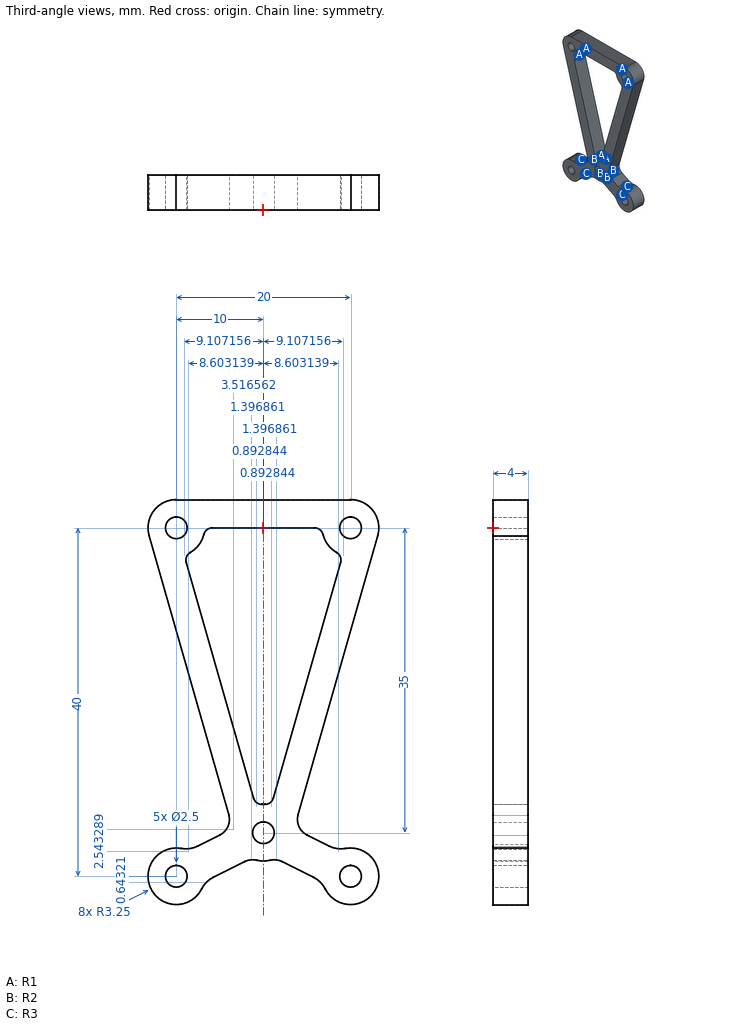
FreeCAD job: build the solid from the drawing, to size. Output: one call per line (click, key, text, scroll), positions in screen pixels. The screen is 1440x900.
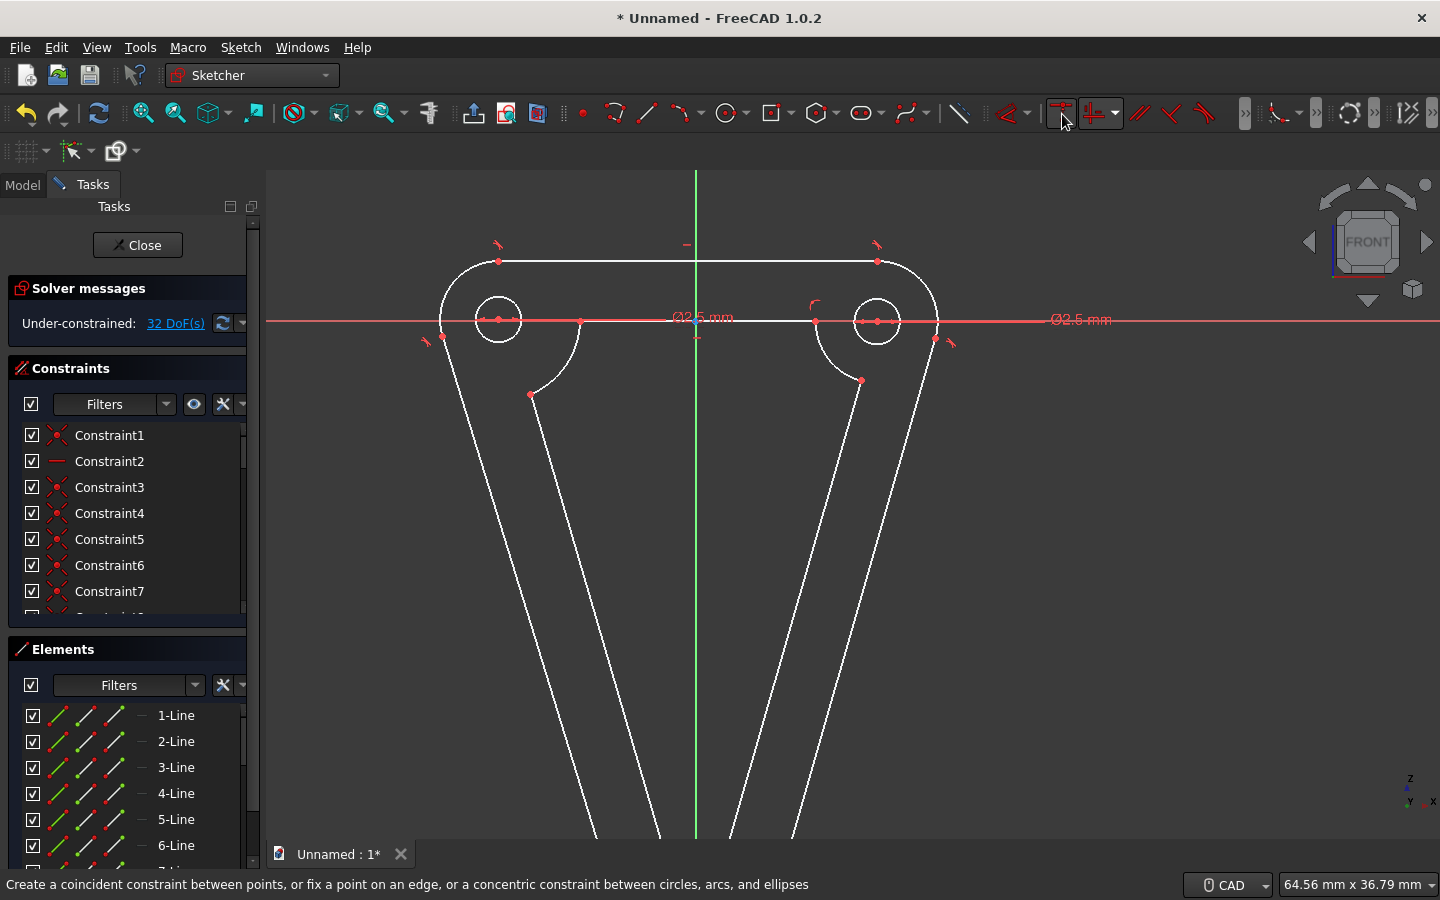
scroll(893, 305, down, 3)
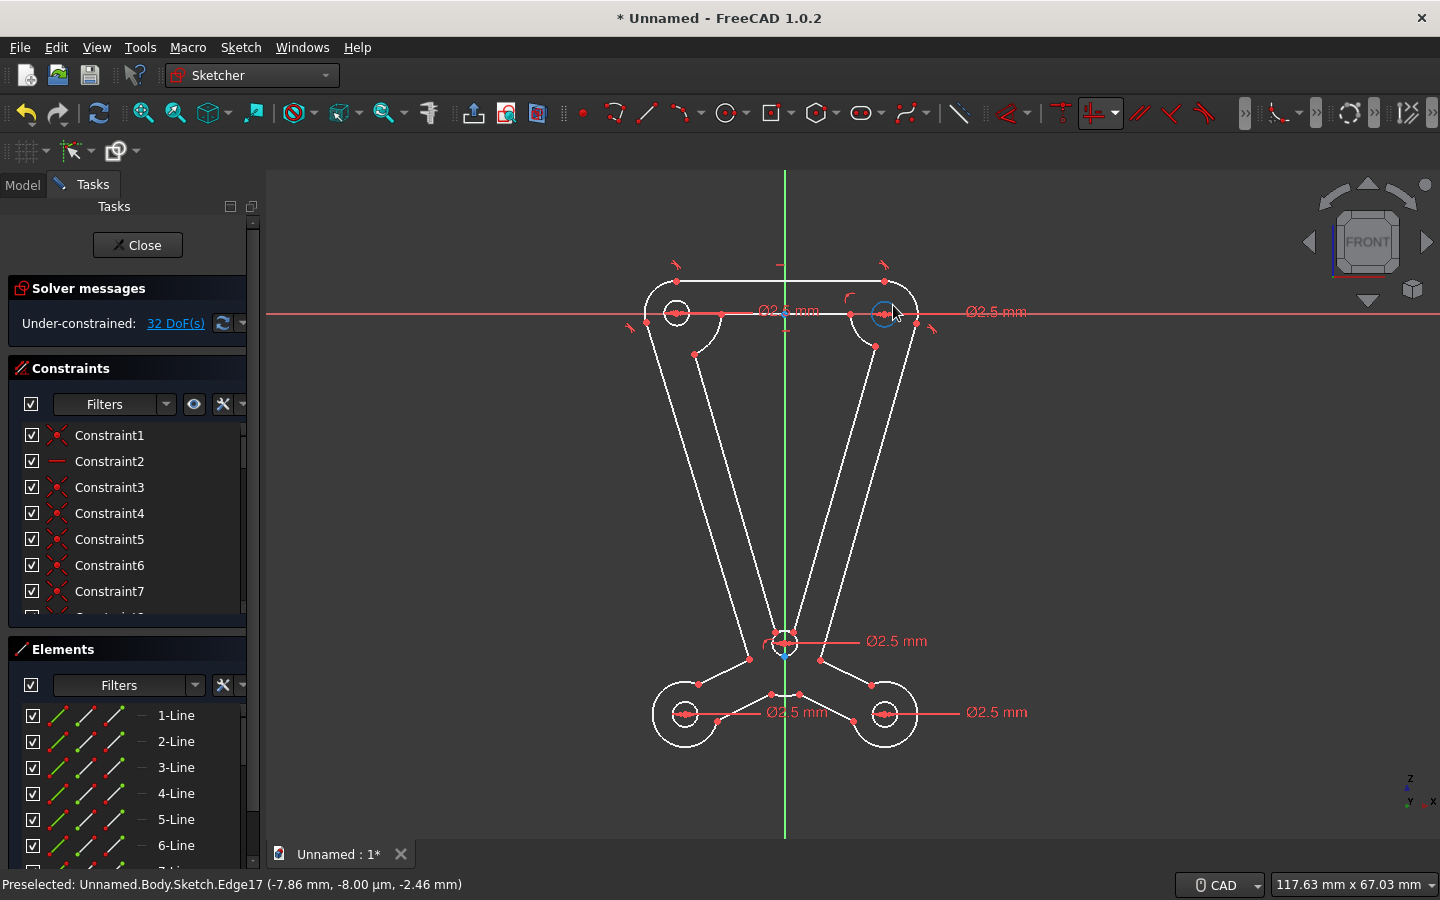
scroll(776, 652, up, 3)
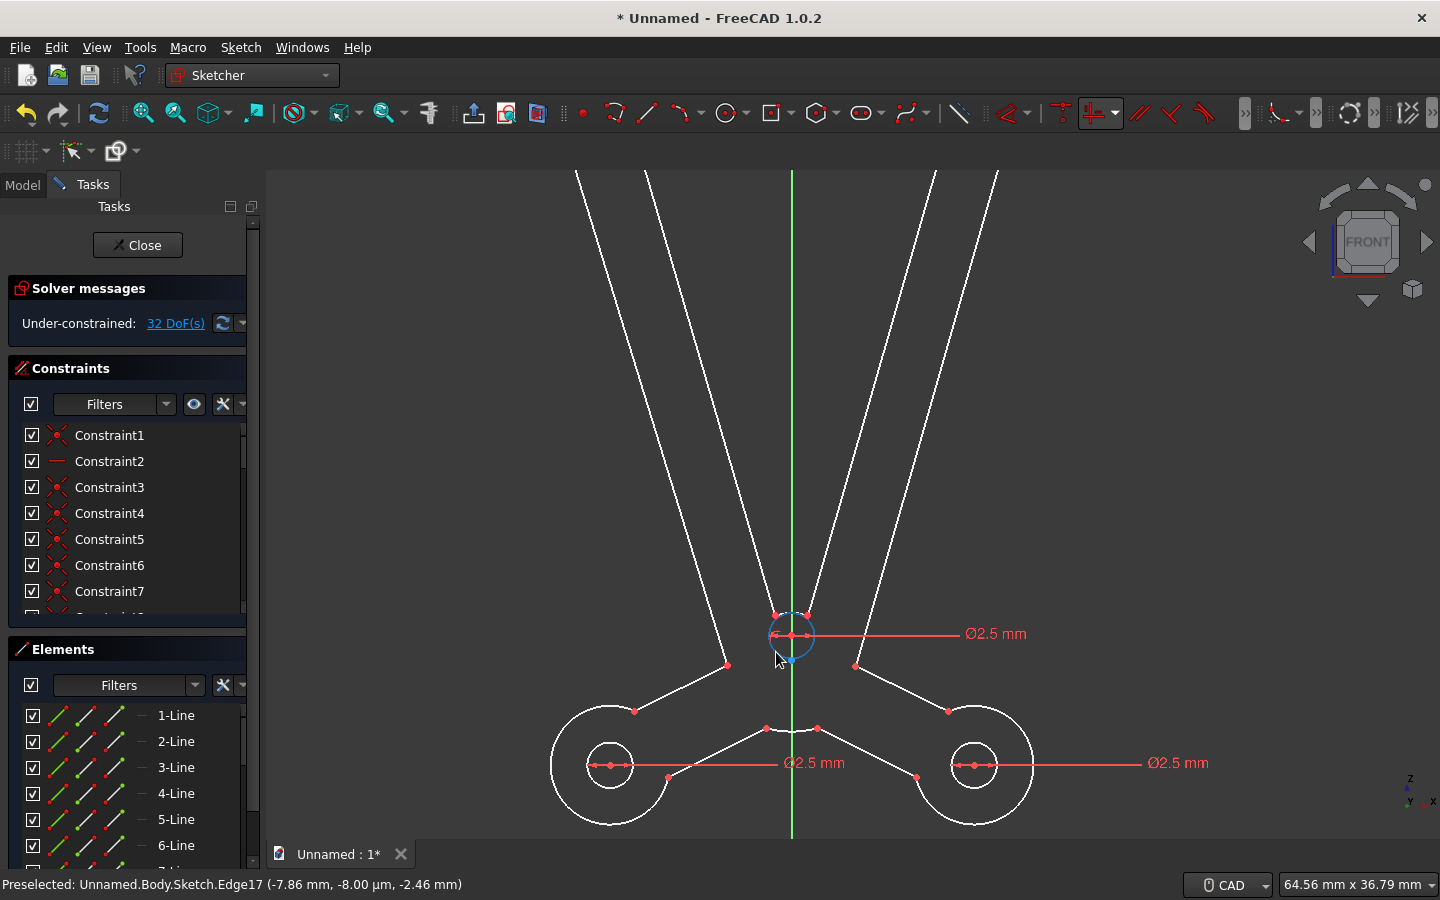
click(776, 652)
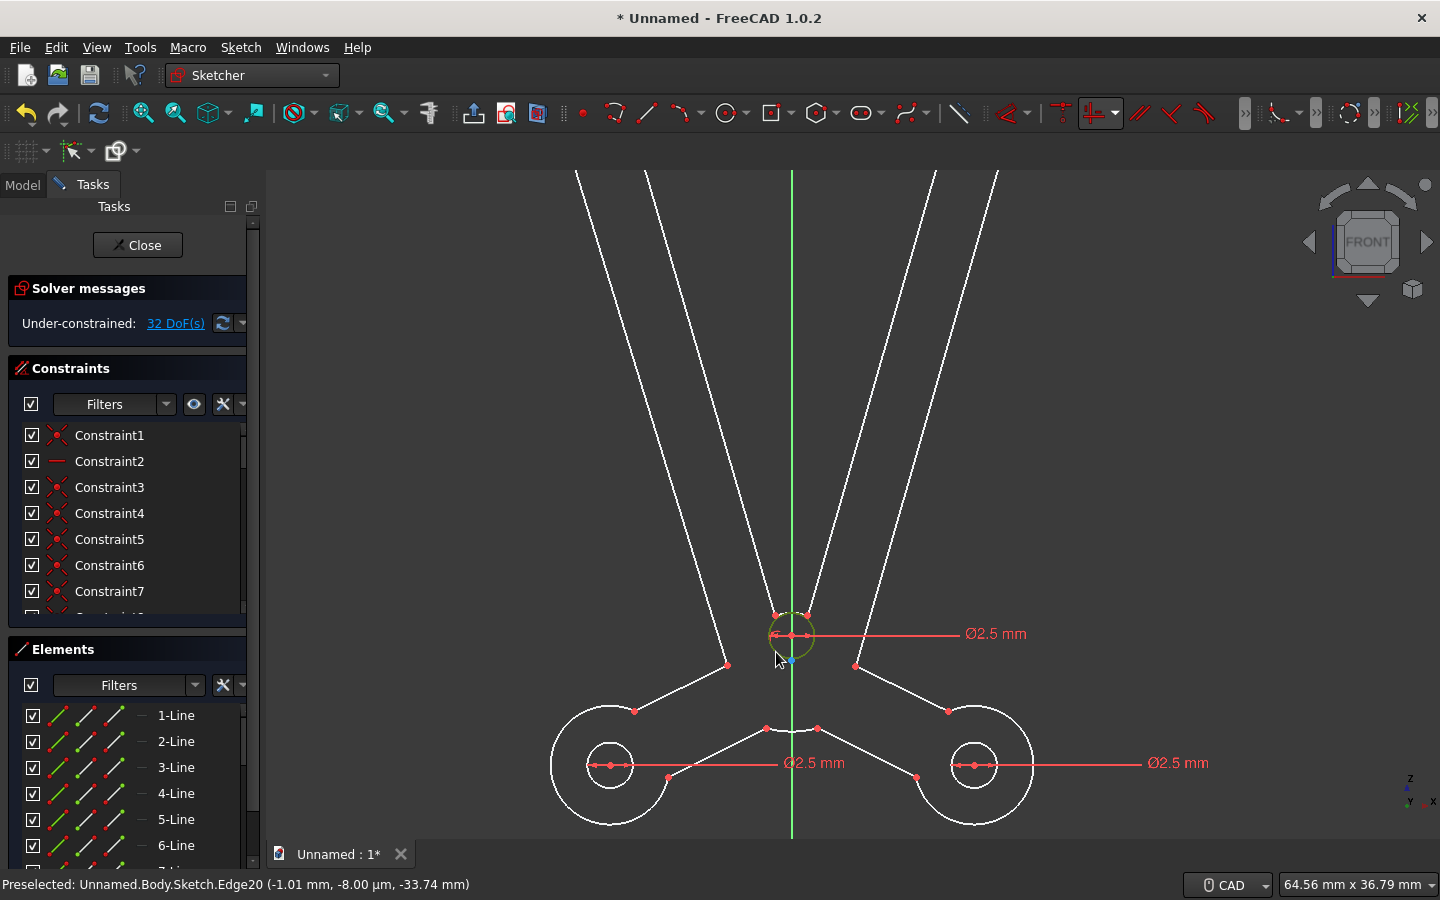
scroll(782, 614, up, 11)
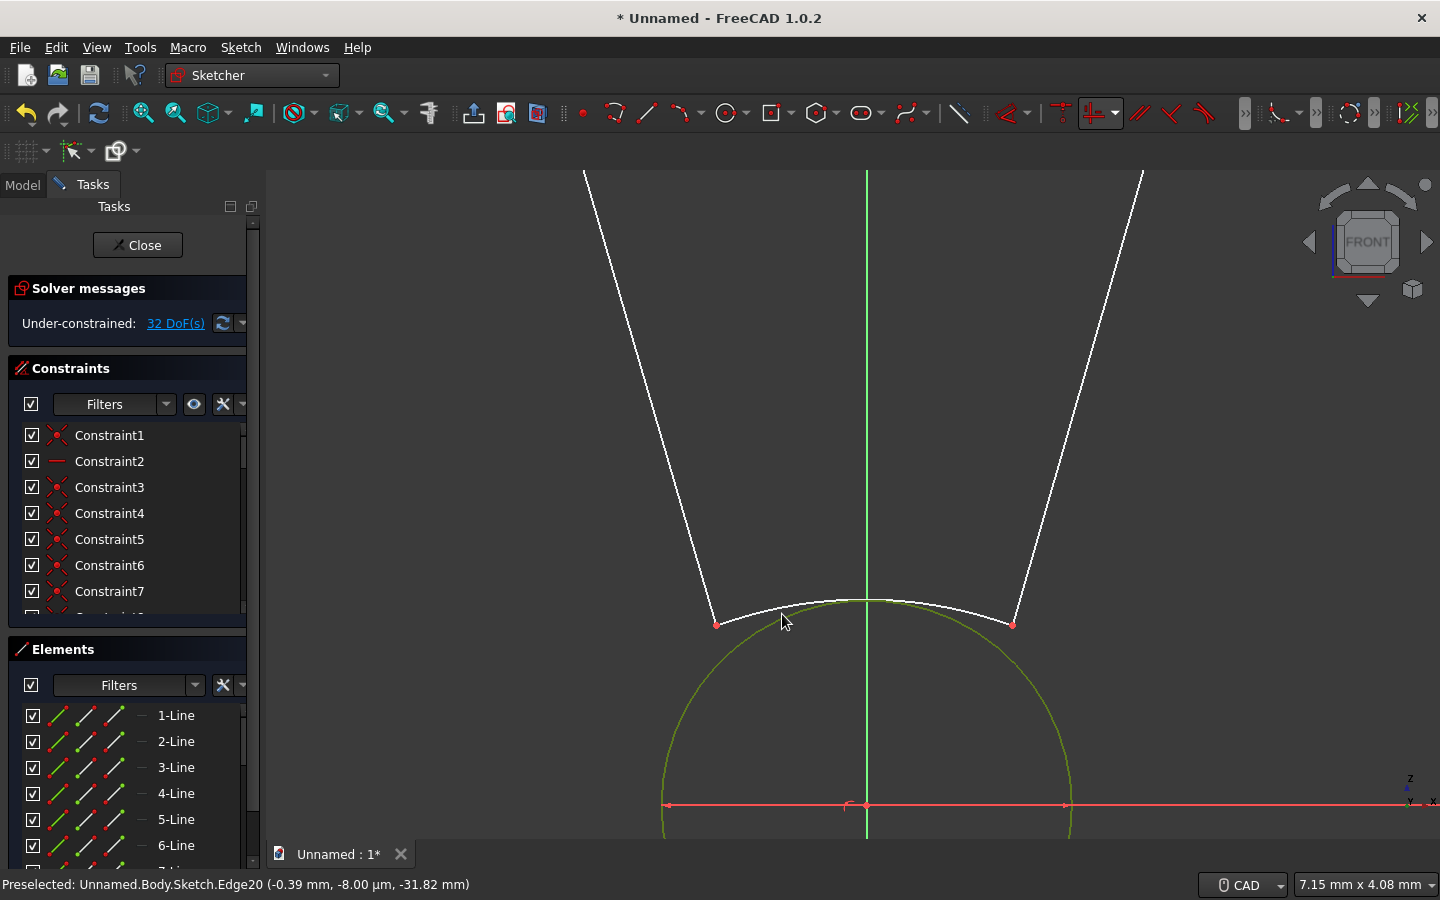
click(774, 609)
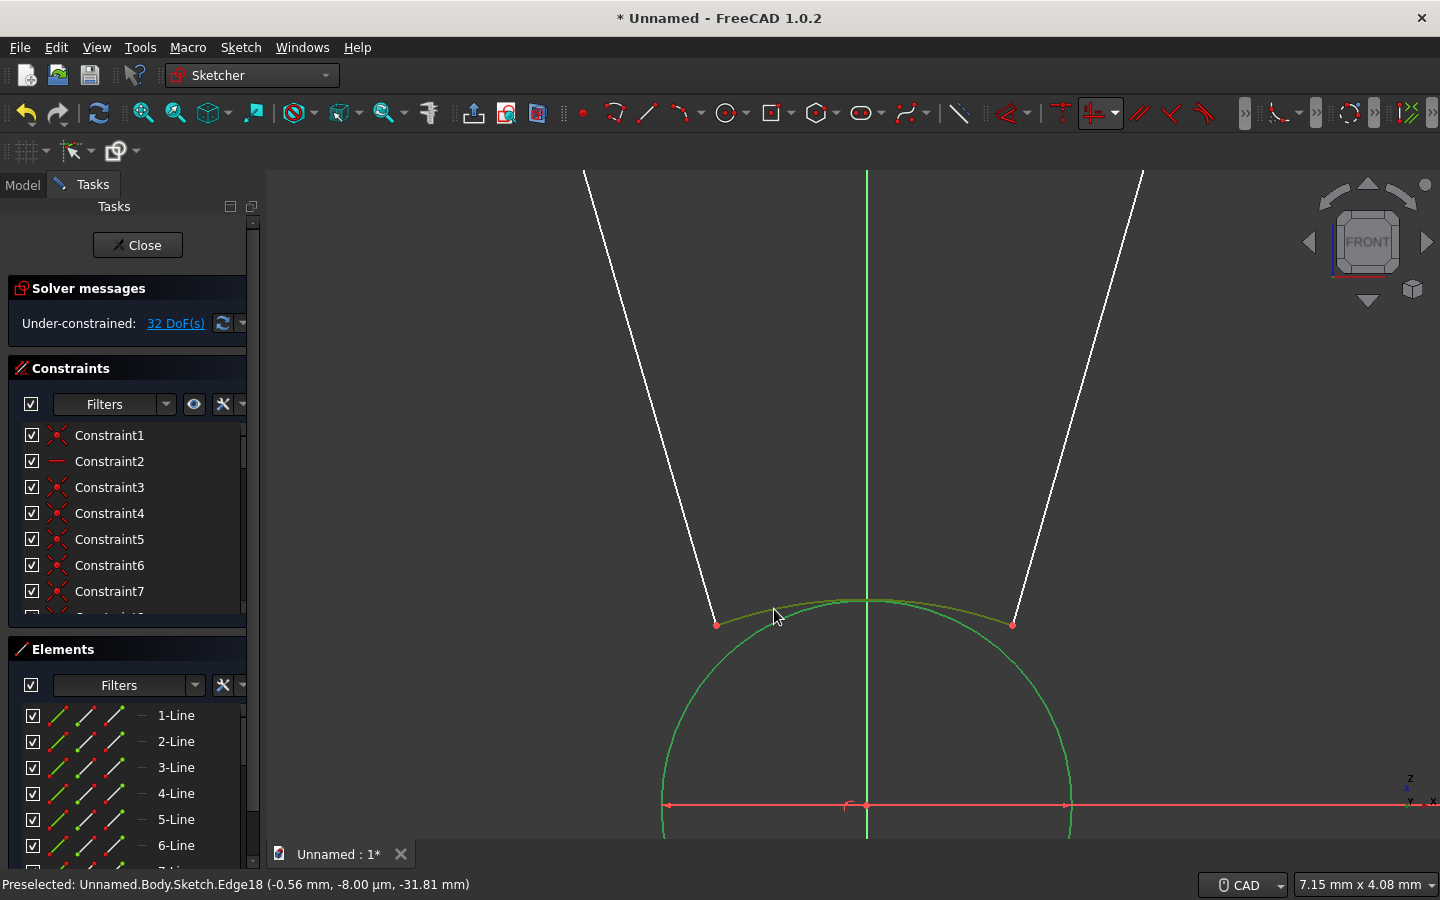
click(1062, 114)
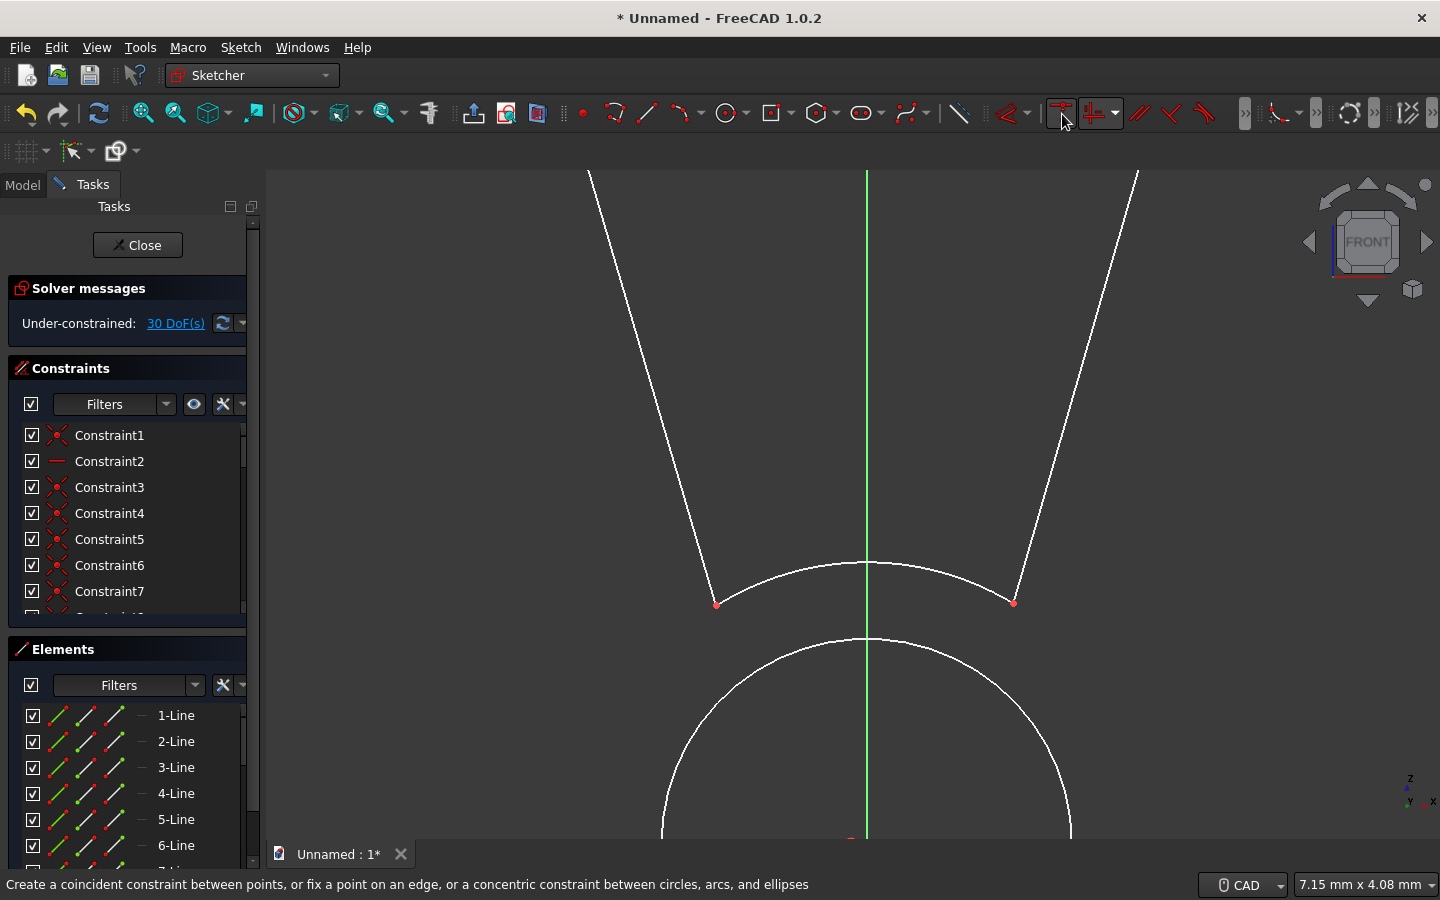
scroll(779, 633, down, 14)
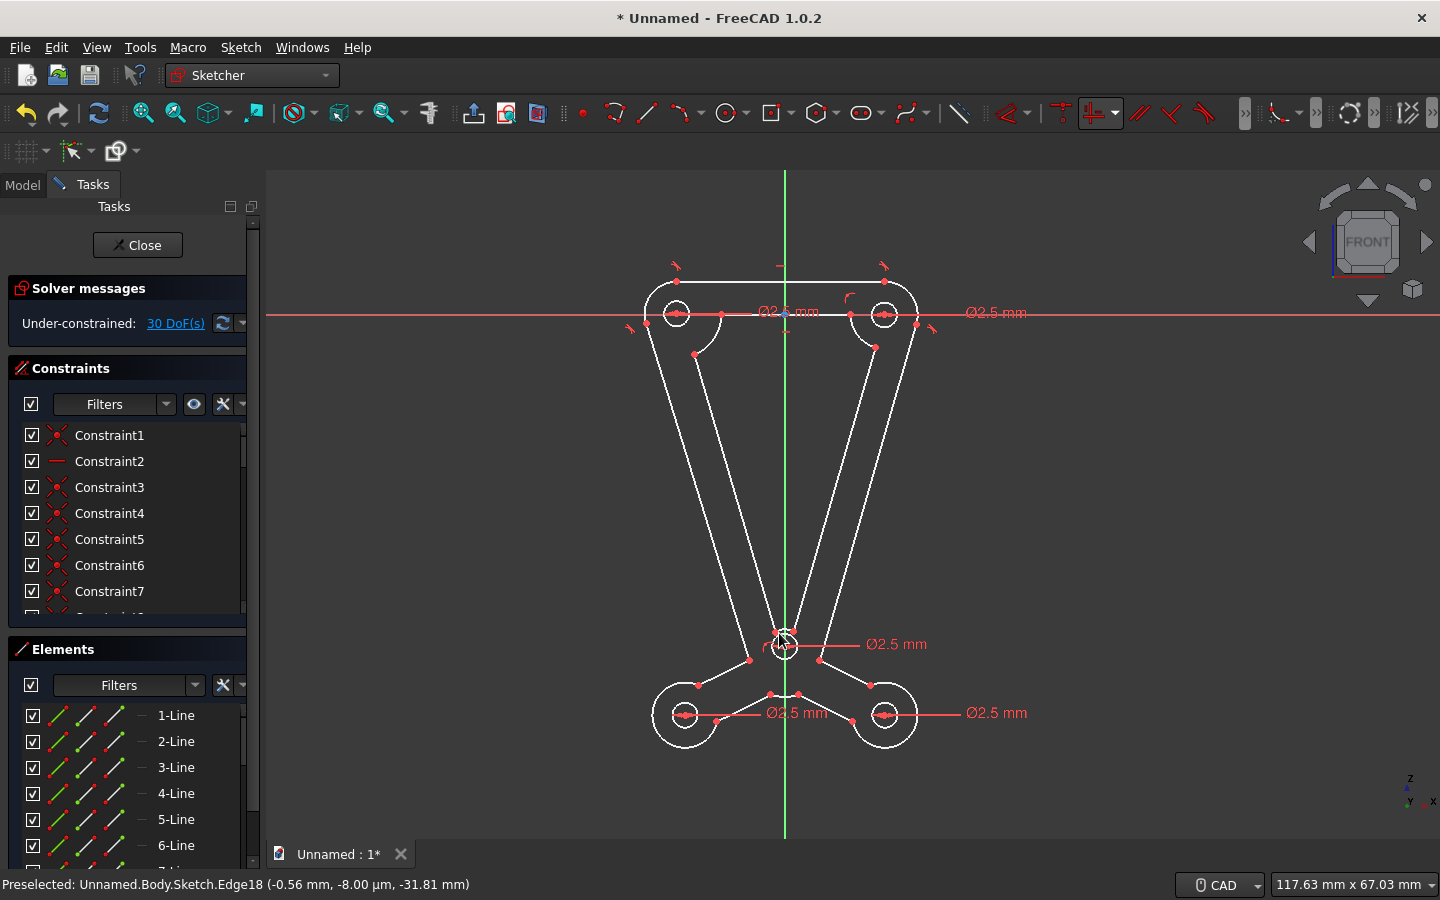
click(660, 287)